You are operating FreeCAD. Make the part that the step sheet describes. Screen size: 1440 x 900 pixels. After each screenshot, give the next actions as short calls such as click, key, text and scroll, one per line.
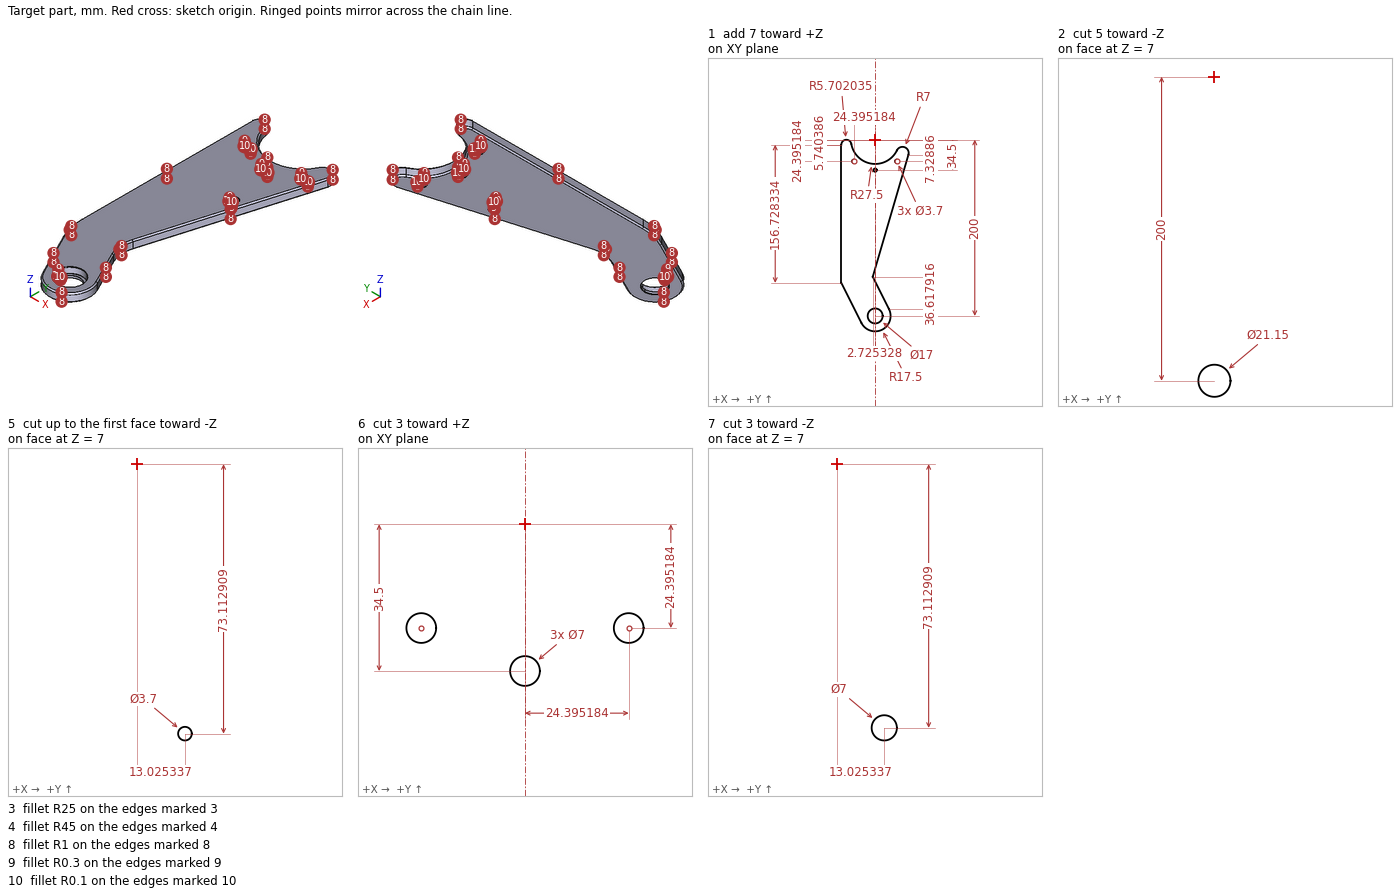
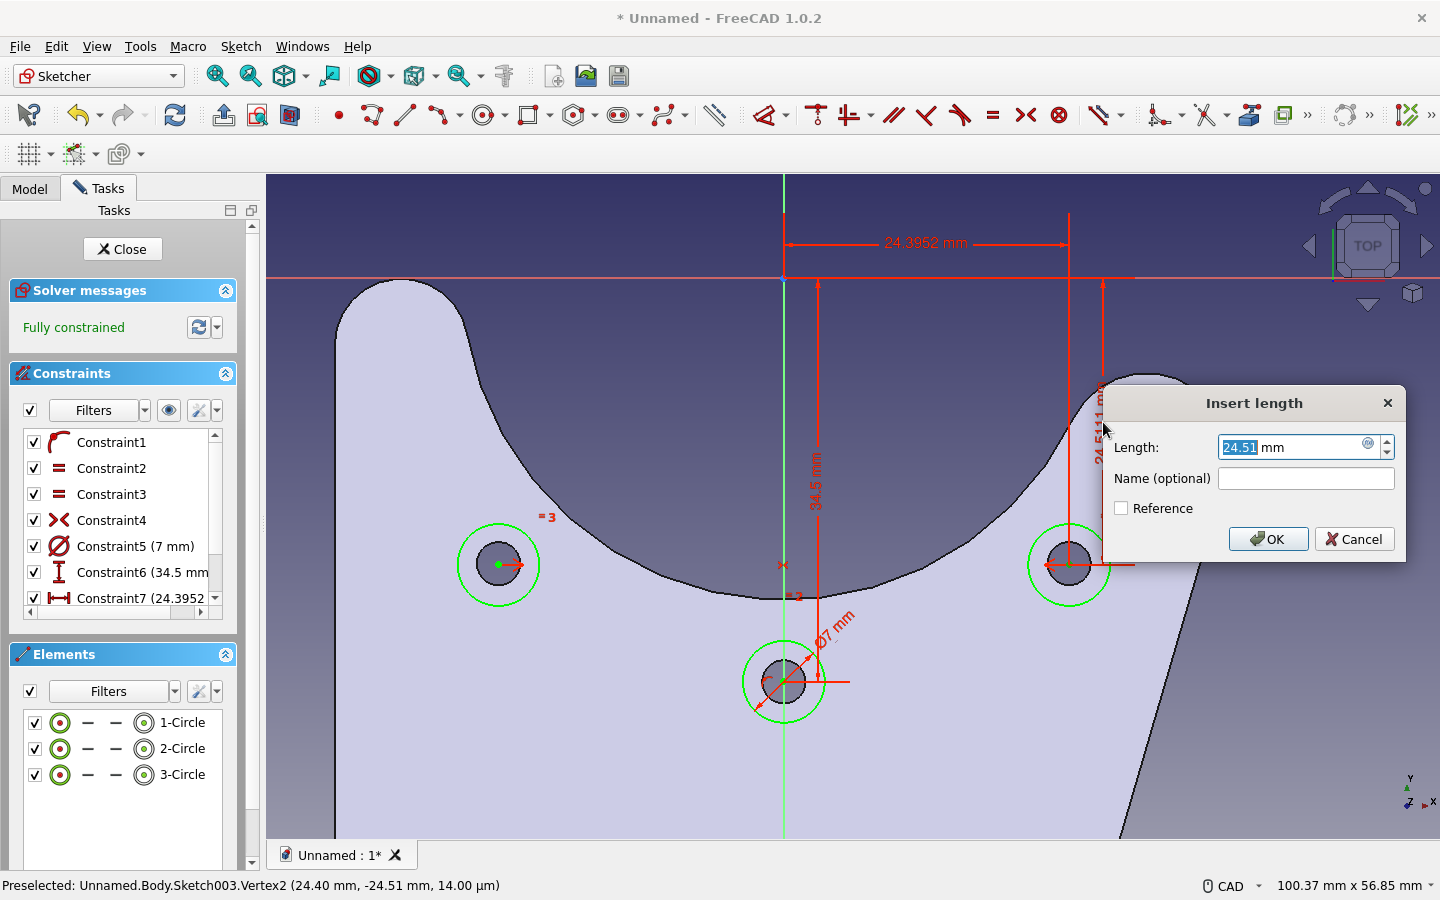
text(24.395184)
key(Return)
key(Escape)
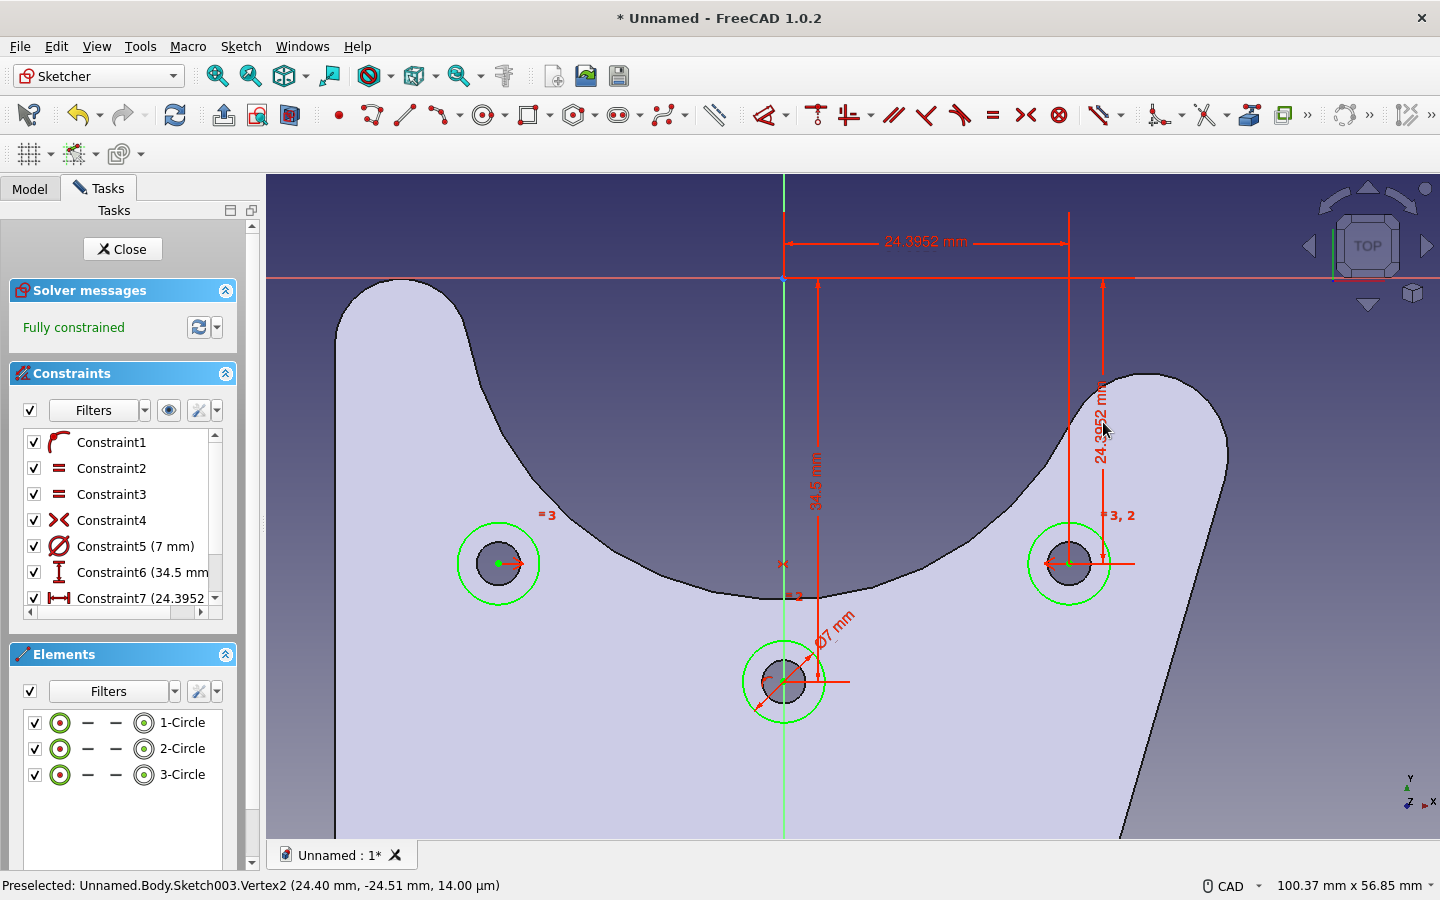
click(123, 249)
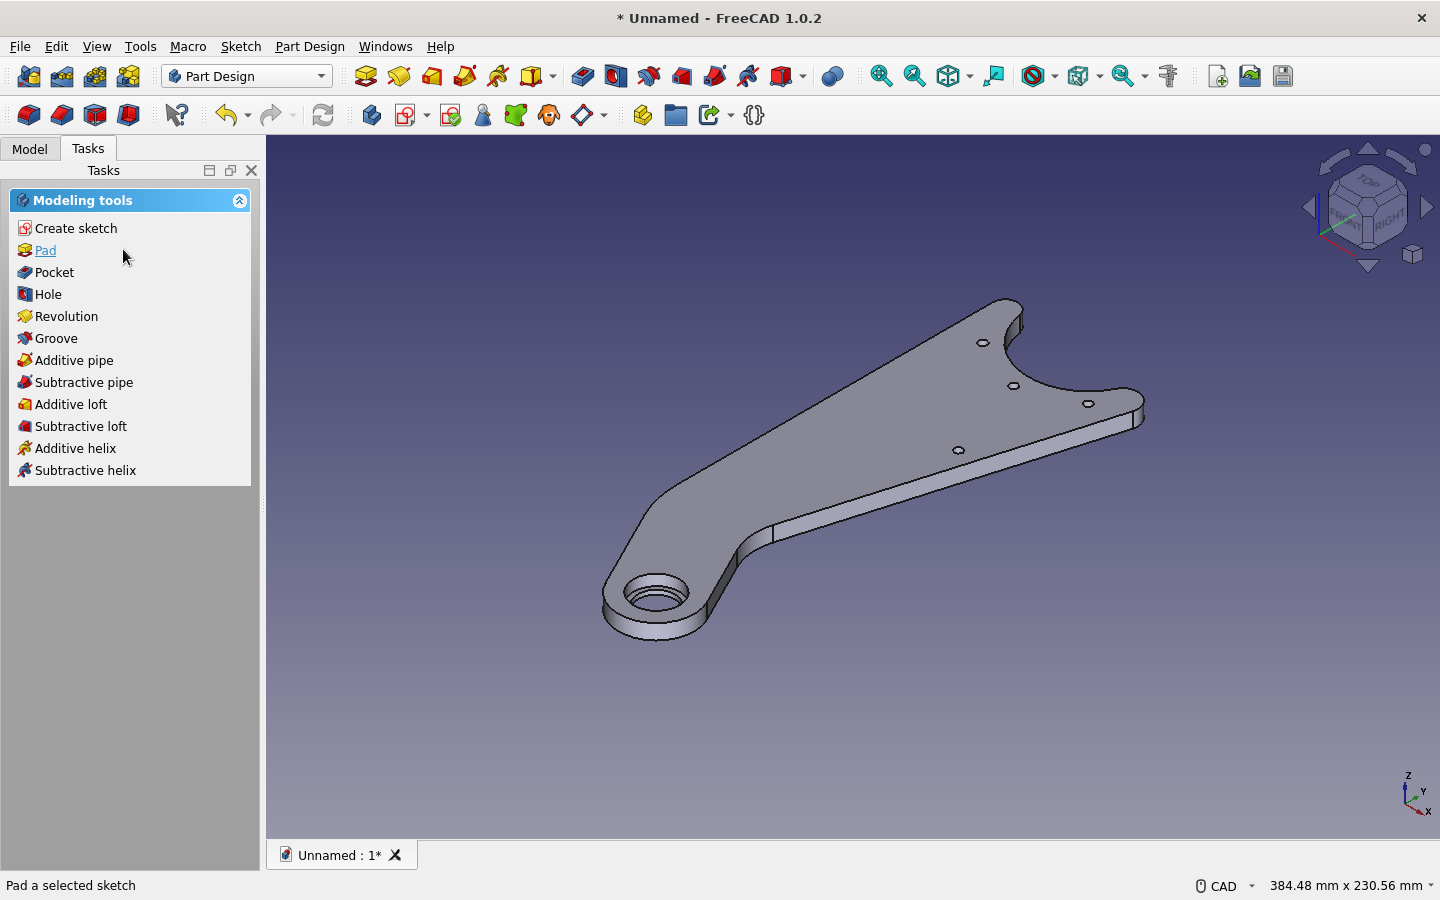
click(583, 76)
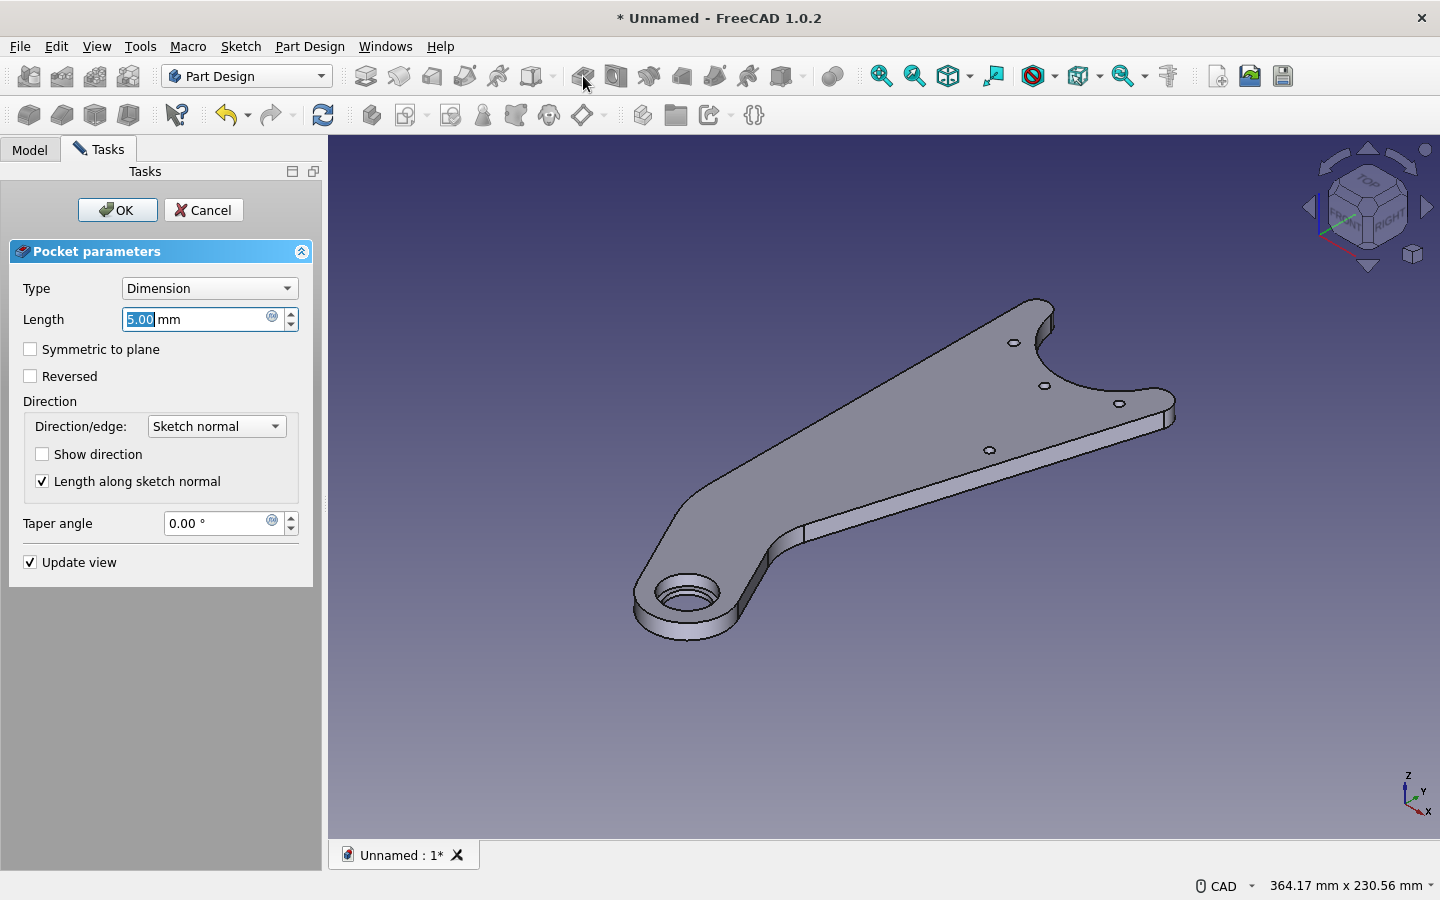
text(3)
key(Tab)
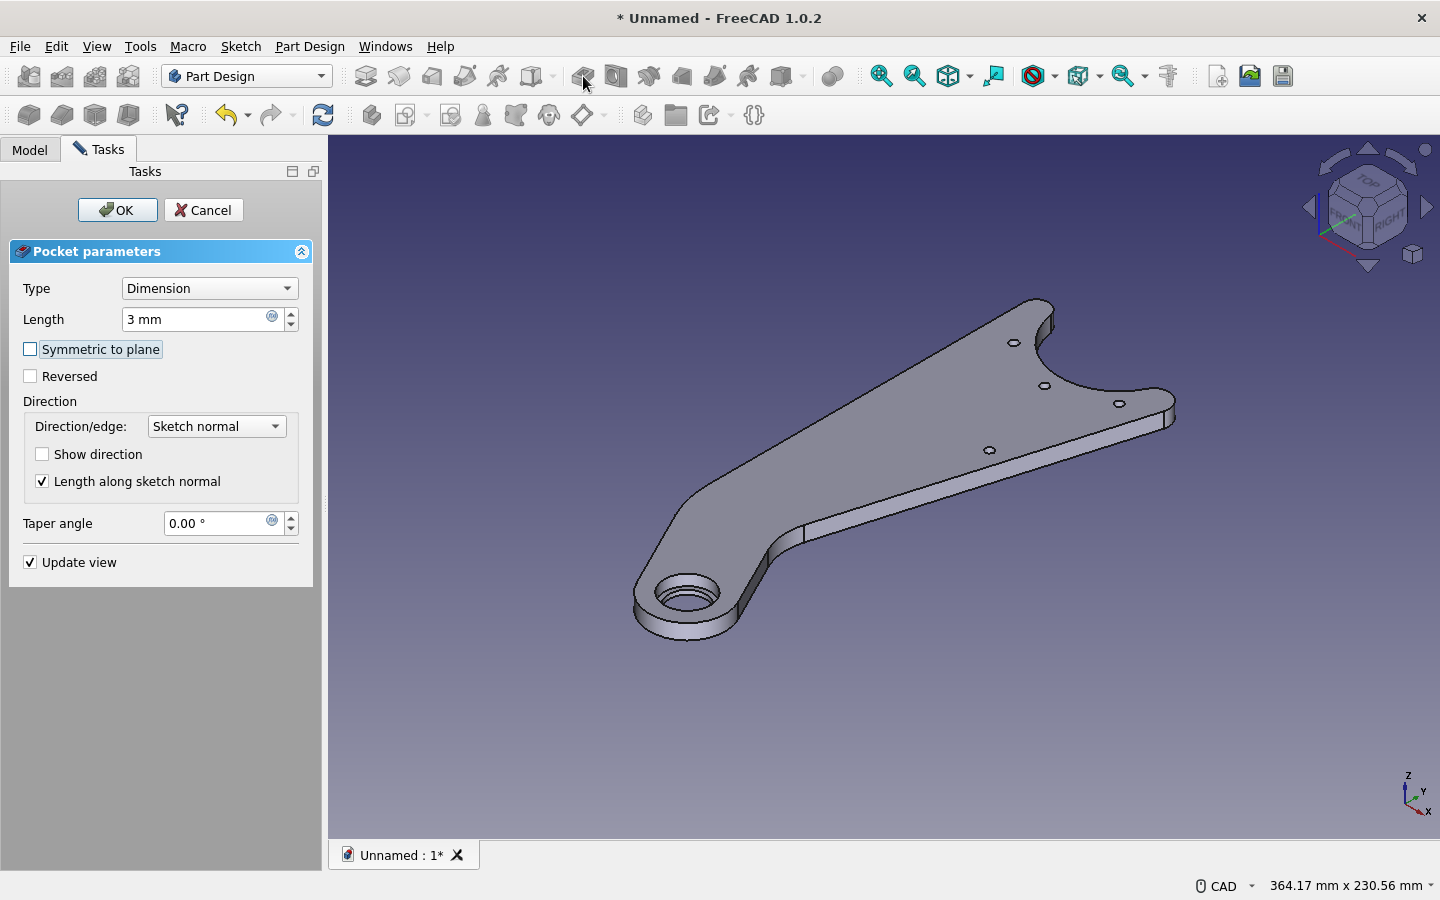
click(31, 376)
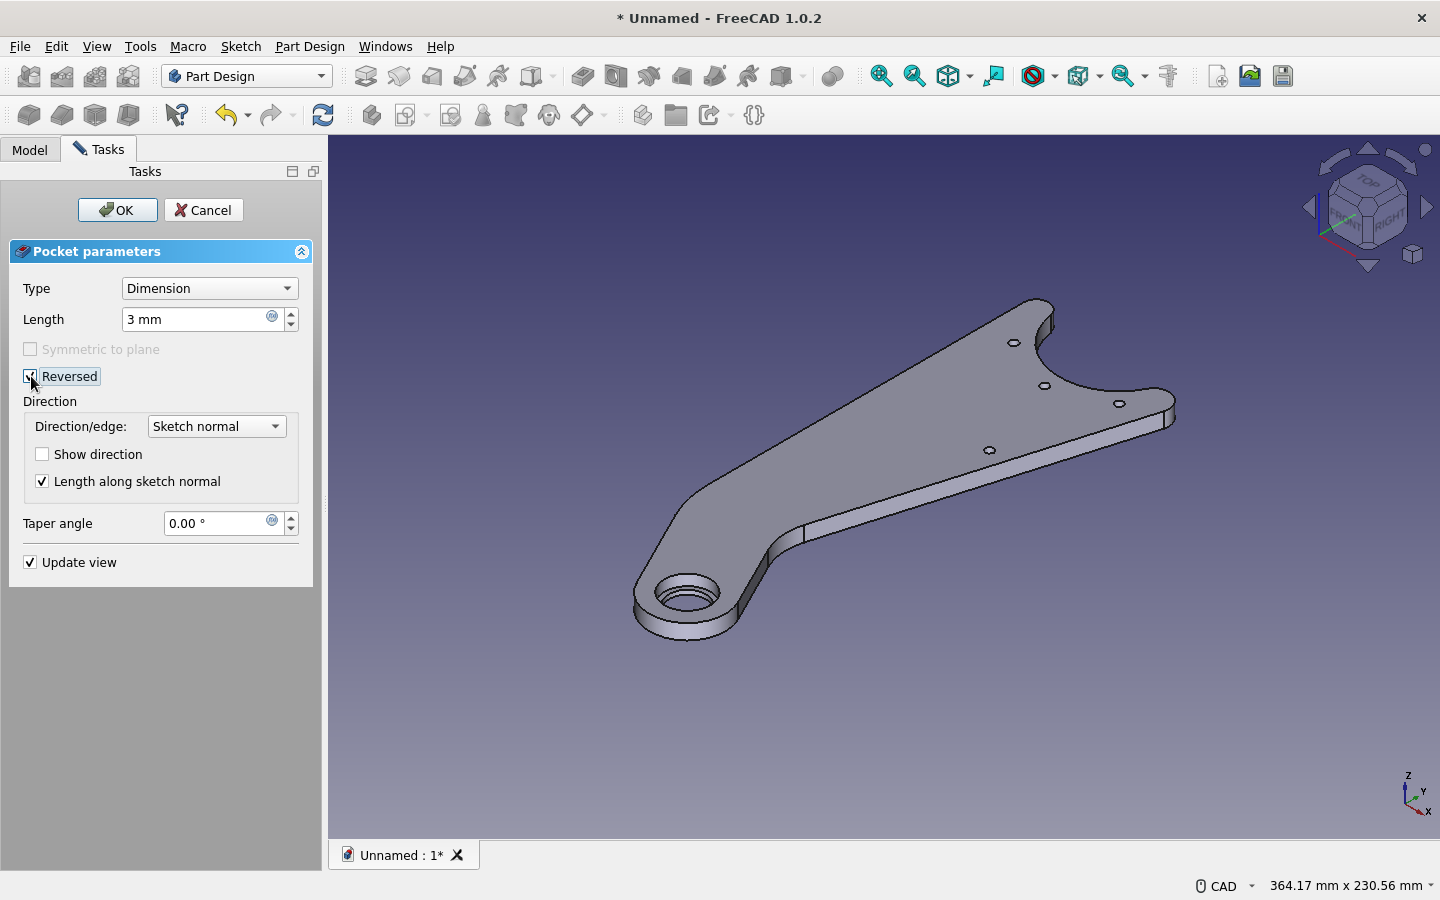
click(118, 210)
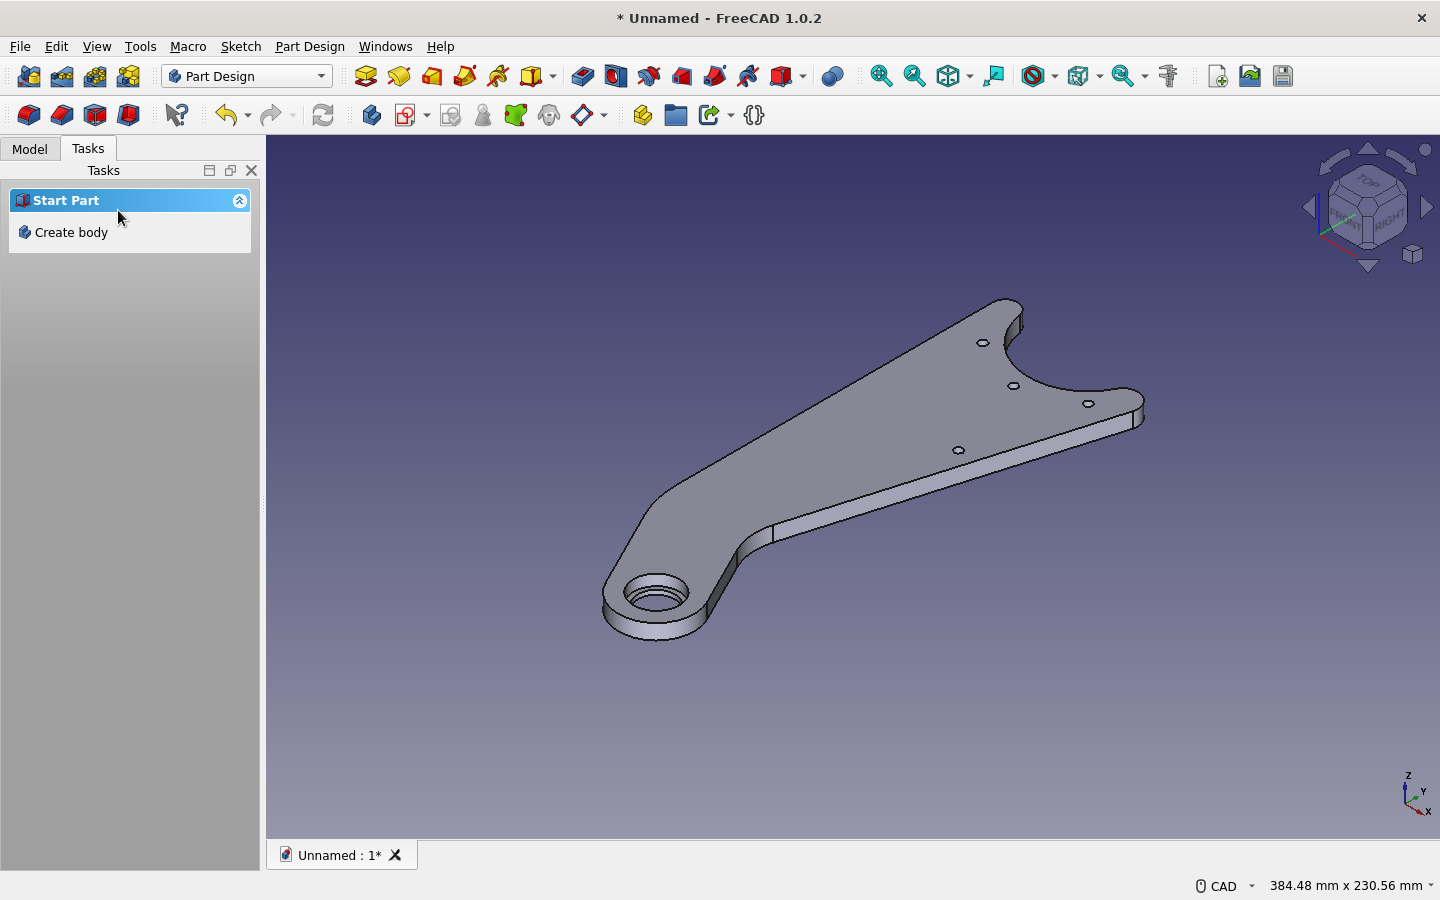
click(896, 425)